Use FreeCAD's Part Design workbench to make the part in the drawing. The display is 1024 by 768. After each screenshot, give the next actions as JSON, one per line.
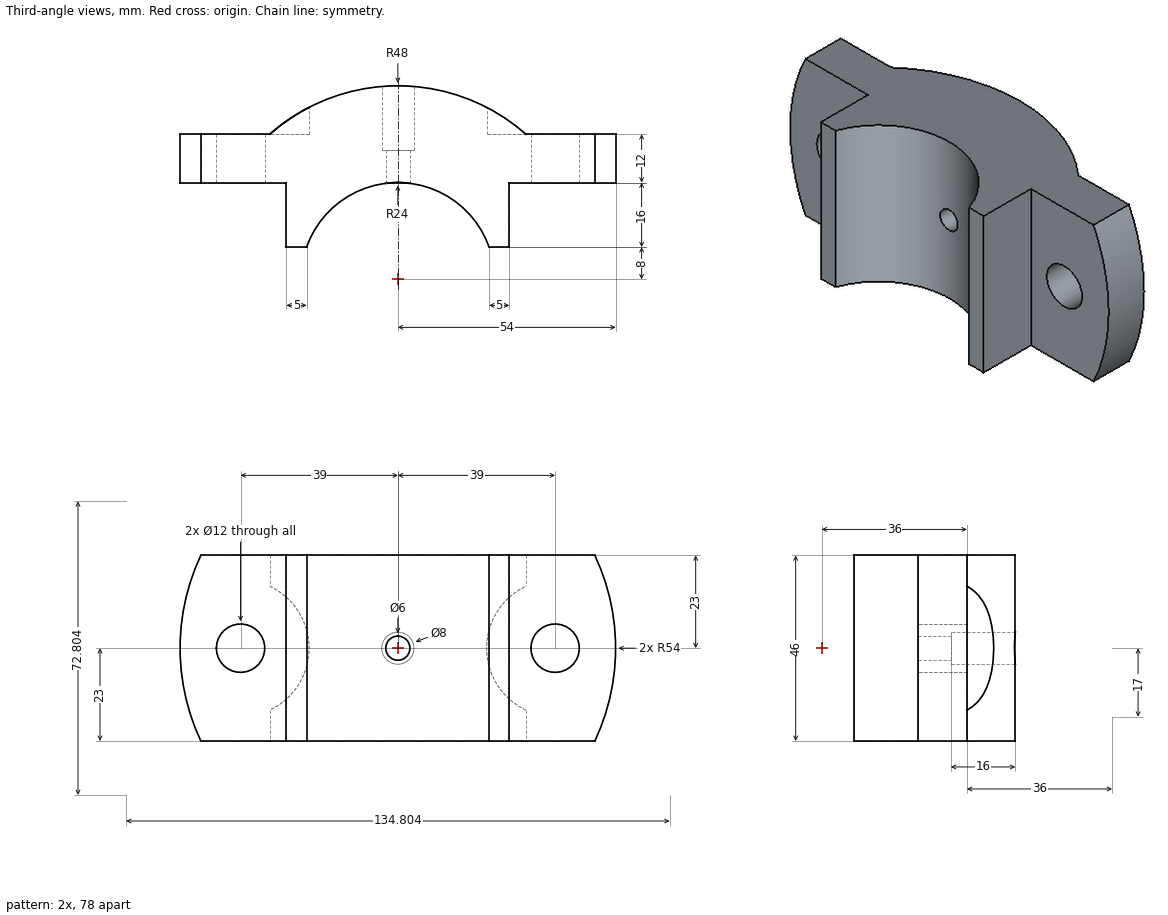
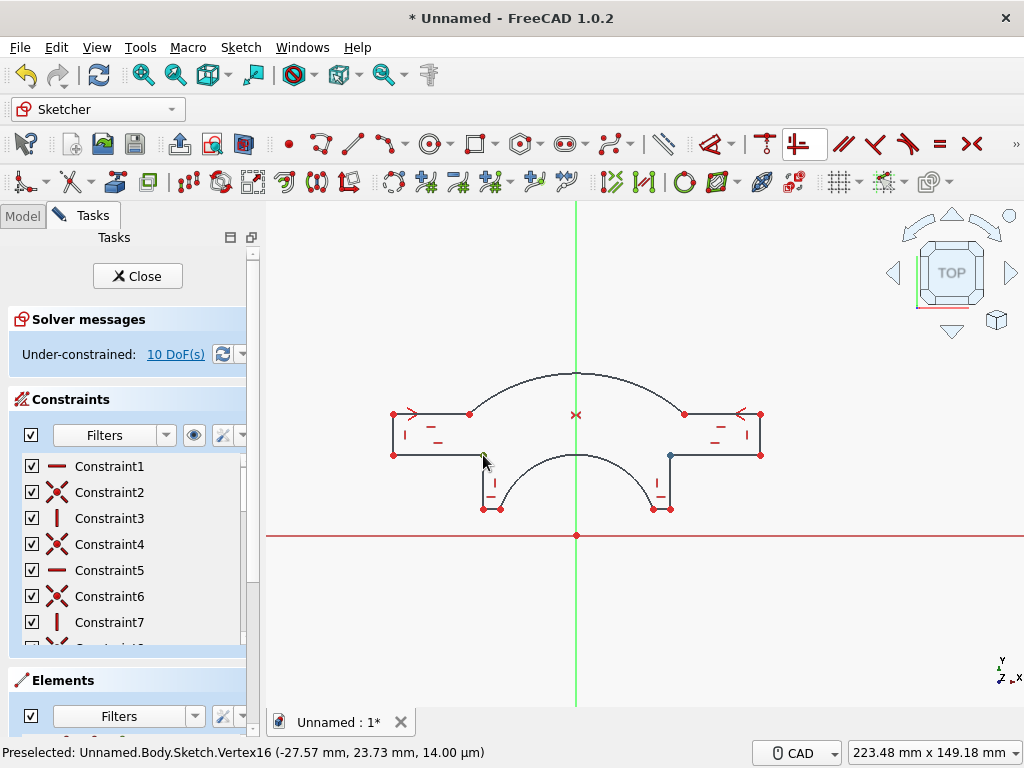
{"action": "left_click", "coordinate": [577, 647]}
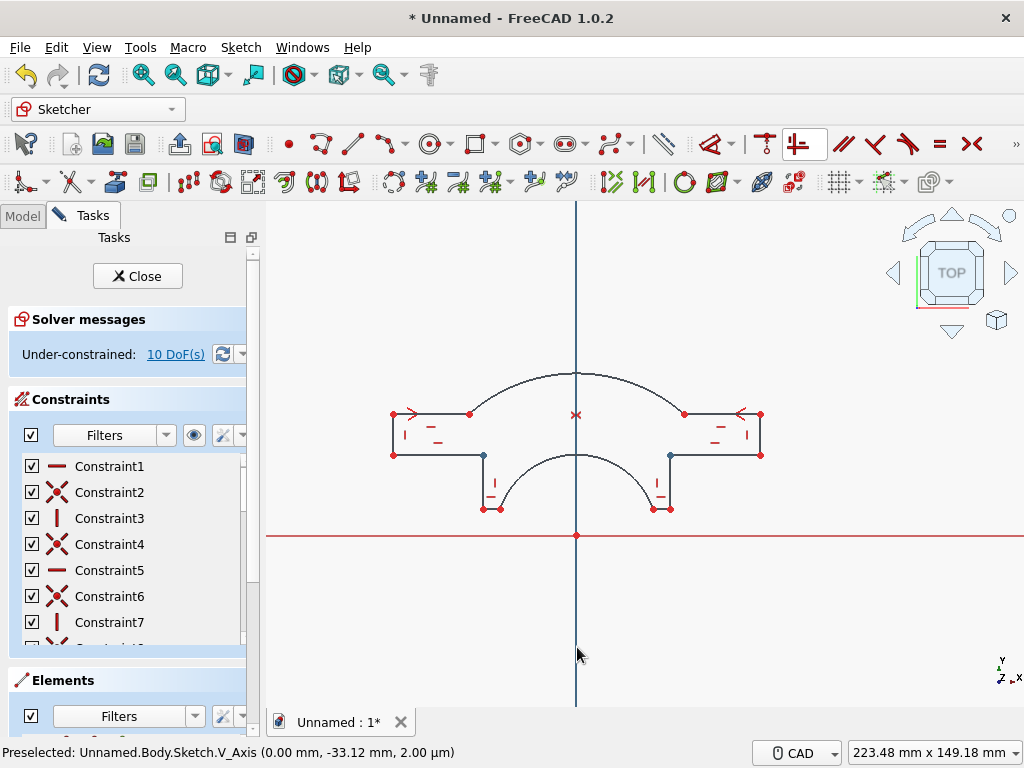
{"action": "left_click", "coordinate": [972, 144]}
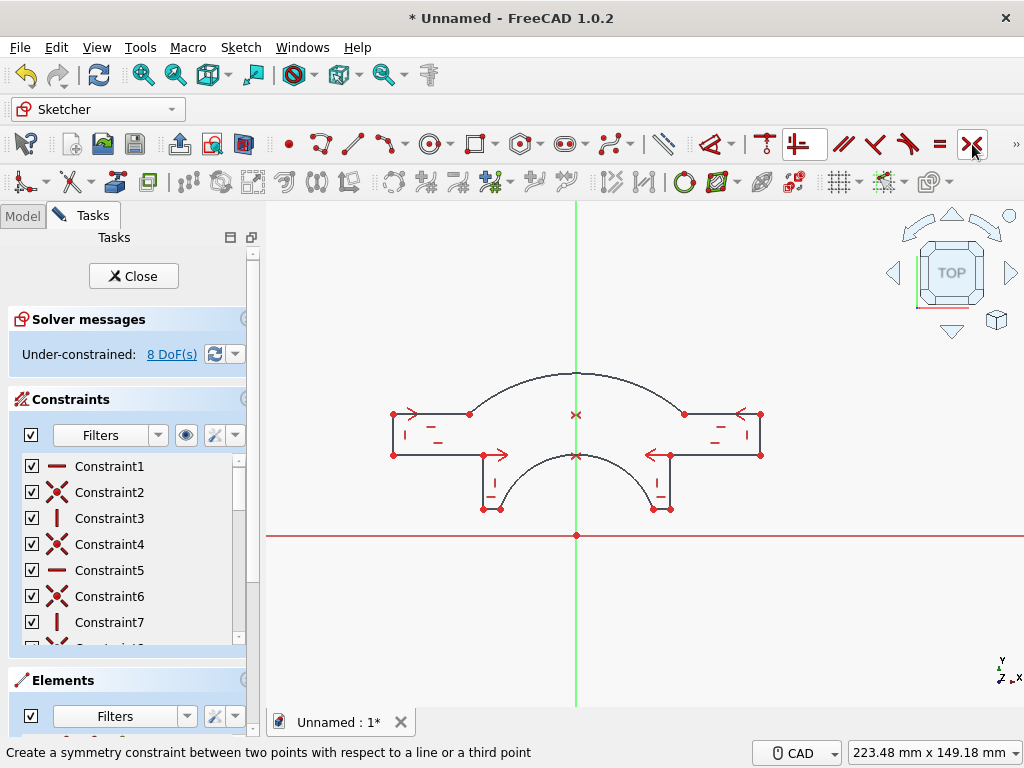
{"action": "left_click", "coordinate": [710, 144]}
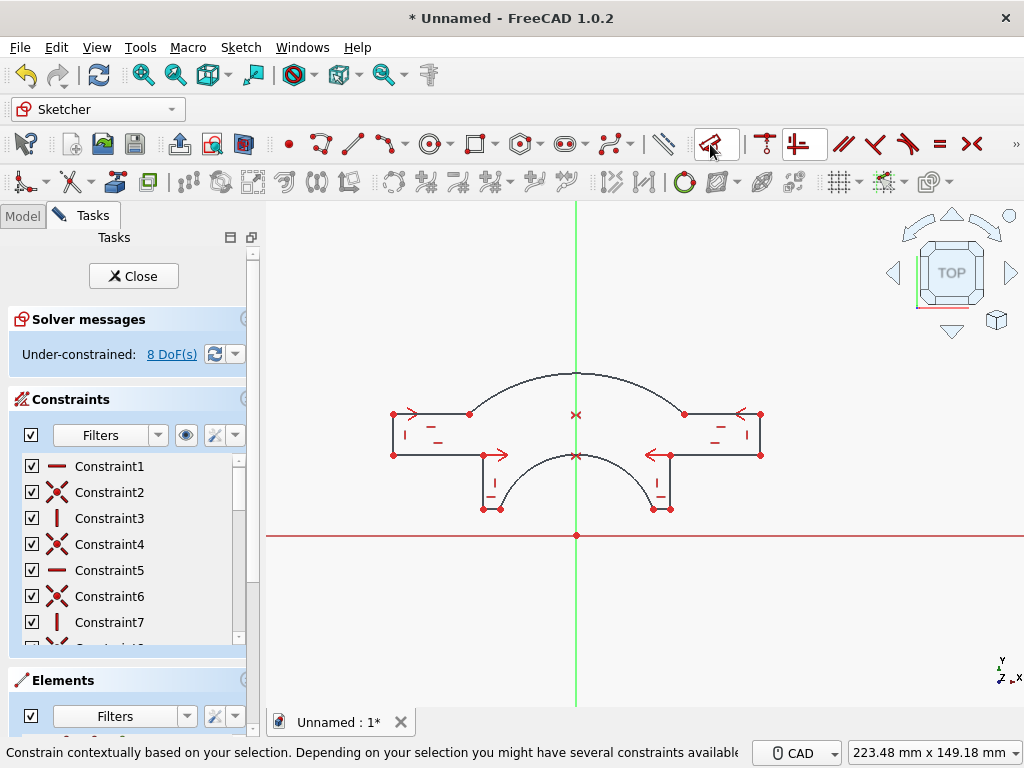
{"action": "left_click", "coordinate": [623, 380]}
{"action": "left_click", "coordinate": [632, 349]}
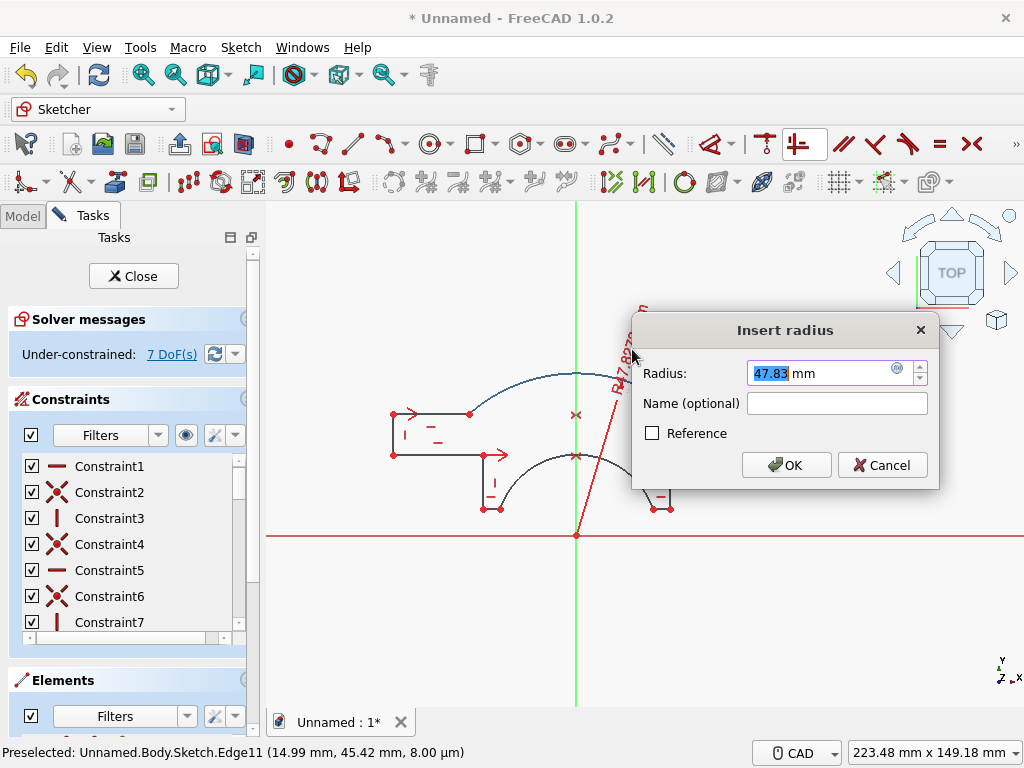
{"action": "type", "text": "48"}
{"action": "key", "text": "Return"}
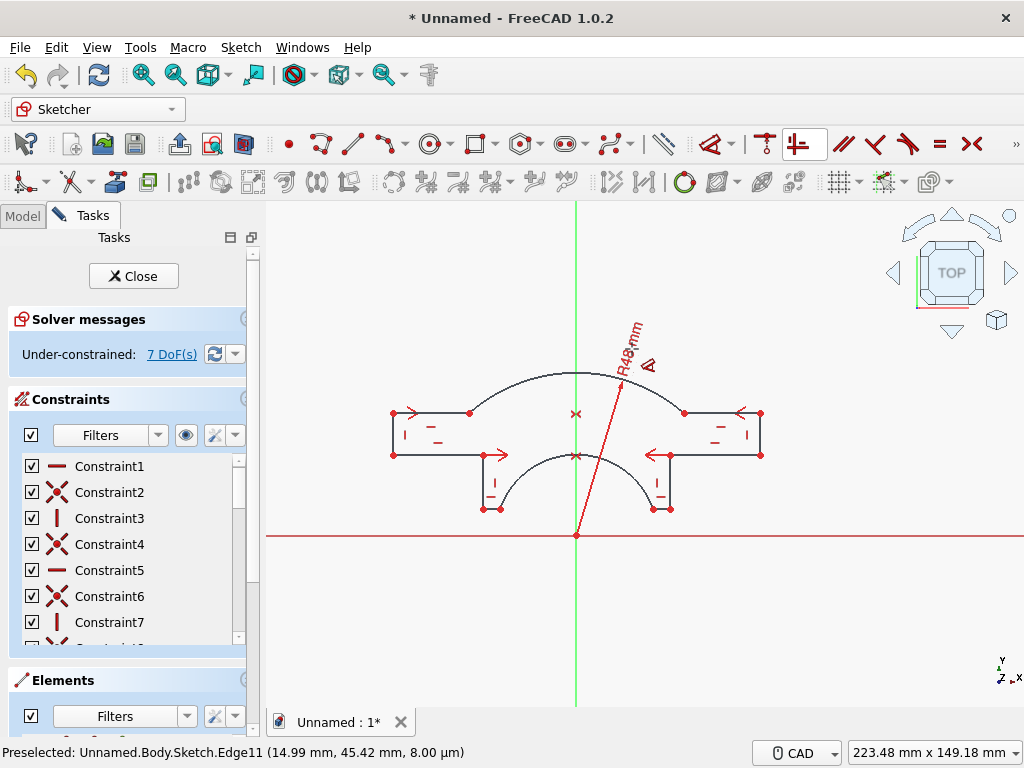
{"action": "left_click", "coordinate": [615, 464]}
{"action": "left_click", "coordinate": [630, 436]}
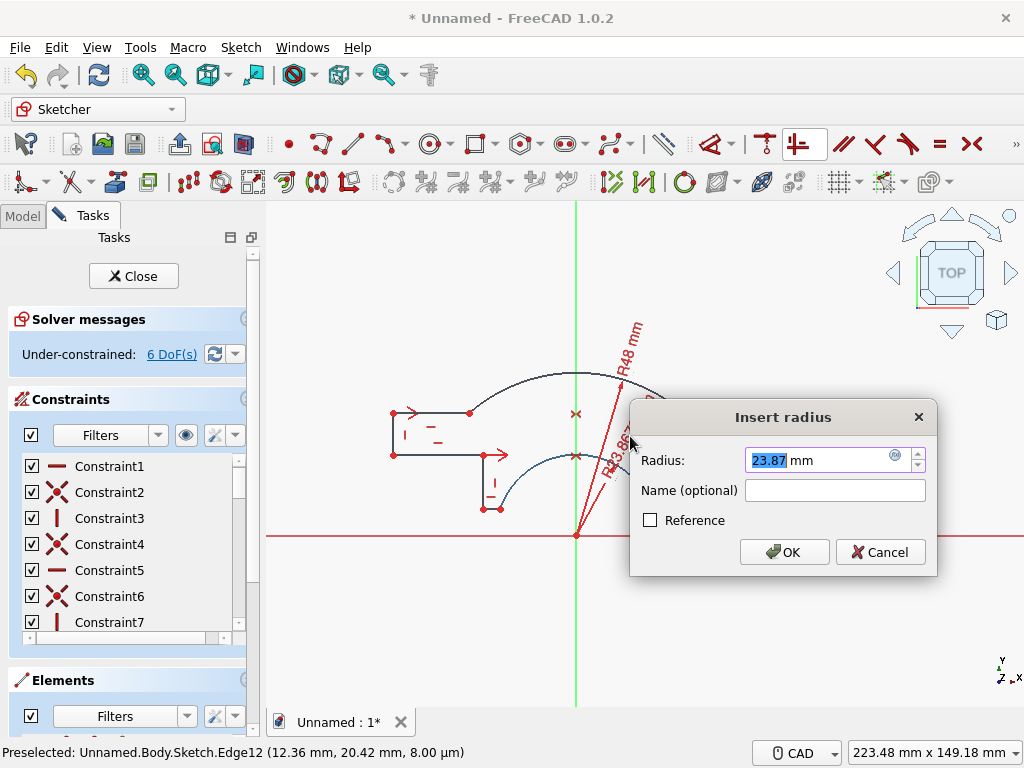
{"action": "type", "text": "24"}
{"action": "key", "text": "Return"}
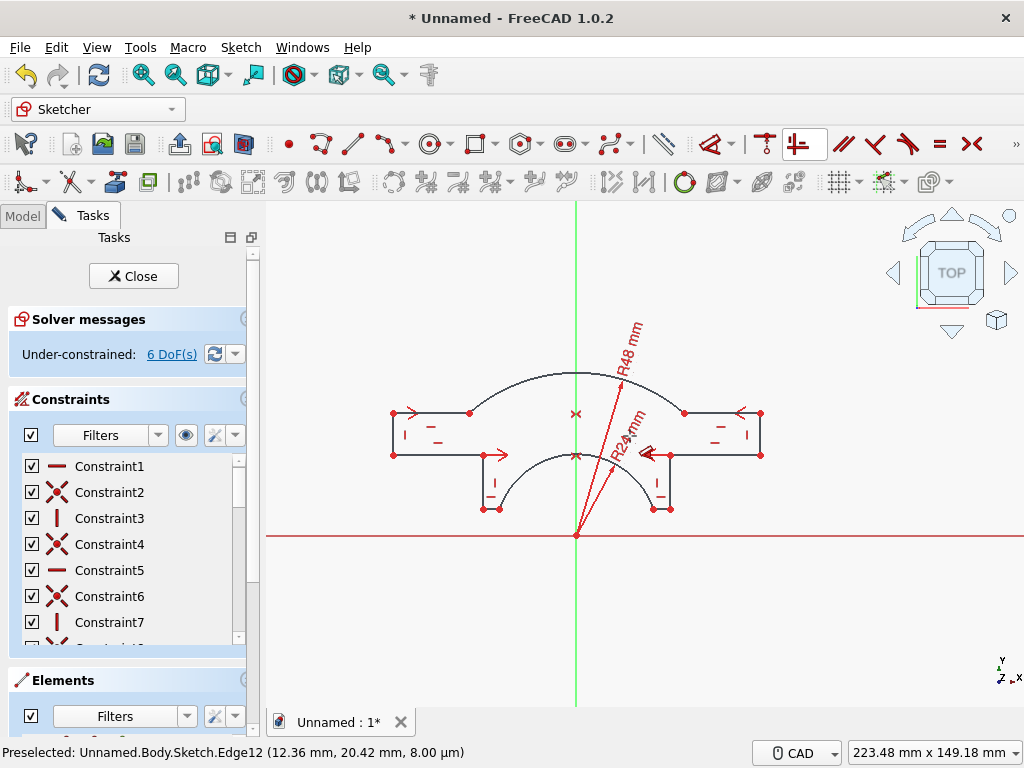
{"action": "scroll", "coordinate": [662, 509], "scroll_direction": "up", "scroll_amount": 5}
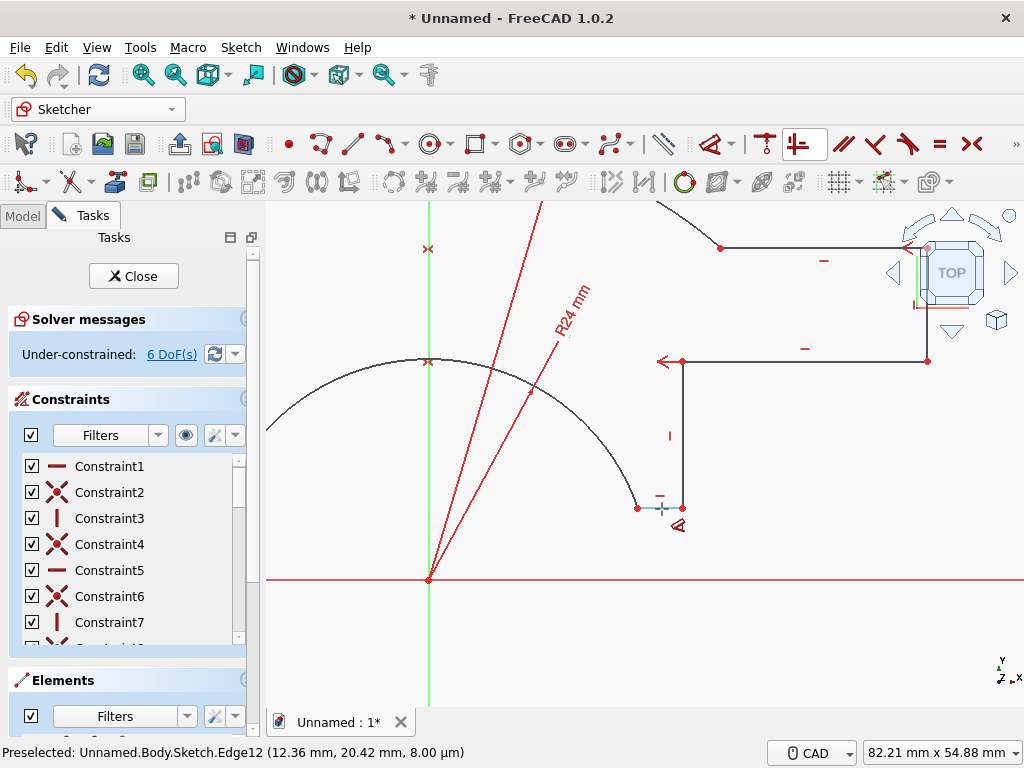
{"action": "left_click", "coordinate": [660, 508]}
{"action": "left_click", "coordinate": [660, 542]}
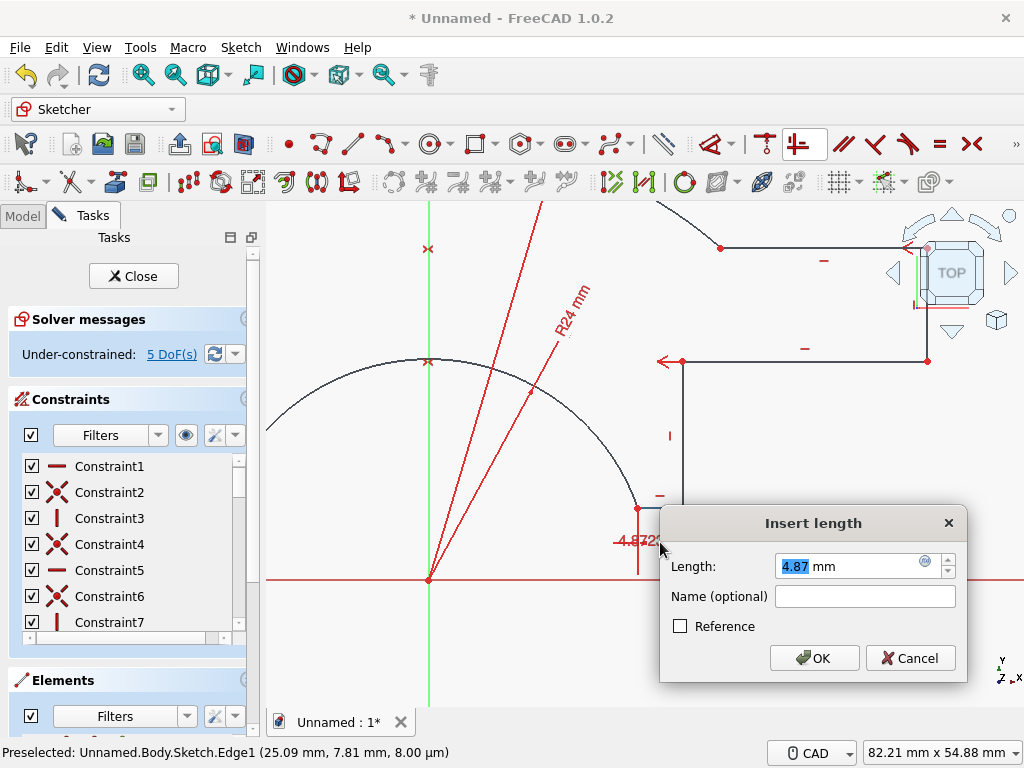
{"action": "type", "text": "5"}
{"action": "key", "text": "Return"}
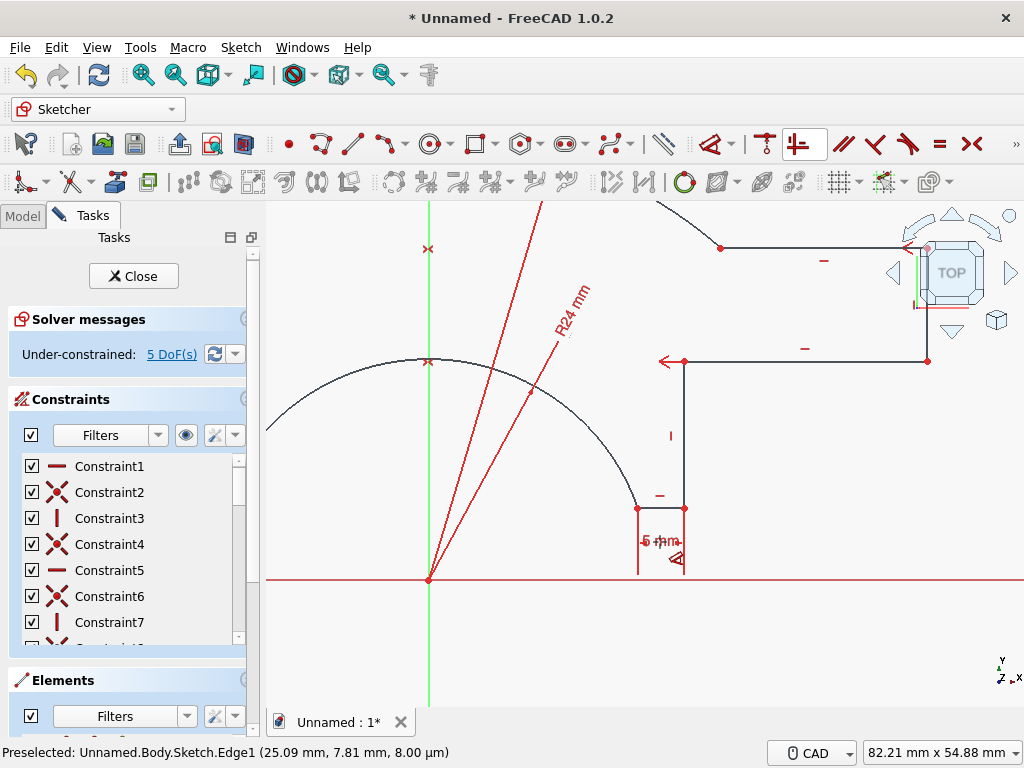
{"action": "scroll", "coordinate": [663, 509], "scroll_direction": "down", "scroll_amount": 5}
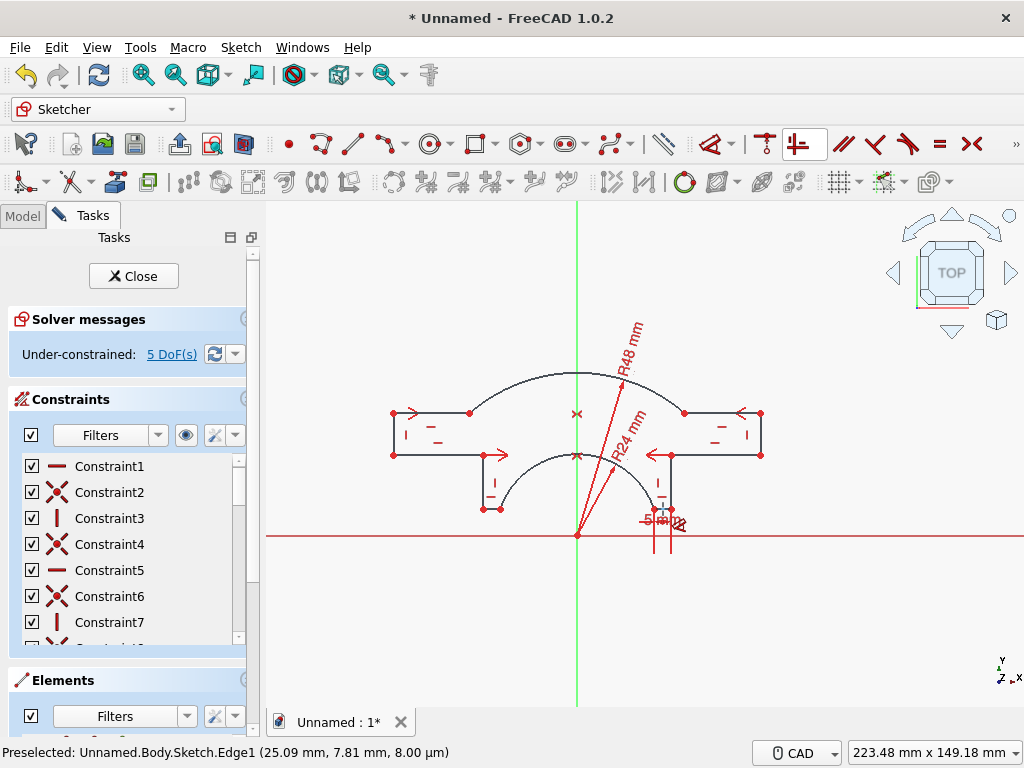
{"action": "scroll", "coordinate": [488, 509], "scroll_direction": "up", "scroll_amount": 5}